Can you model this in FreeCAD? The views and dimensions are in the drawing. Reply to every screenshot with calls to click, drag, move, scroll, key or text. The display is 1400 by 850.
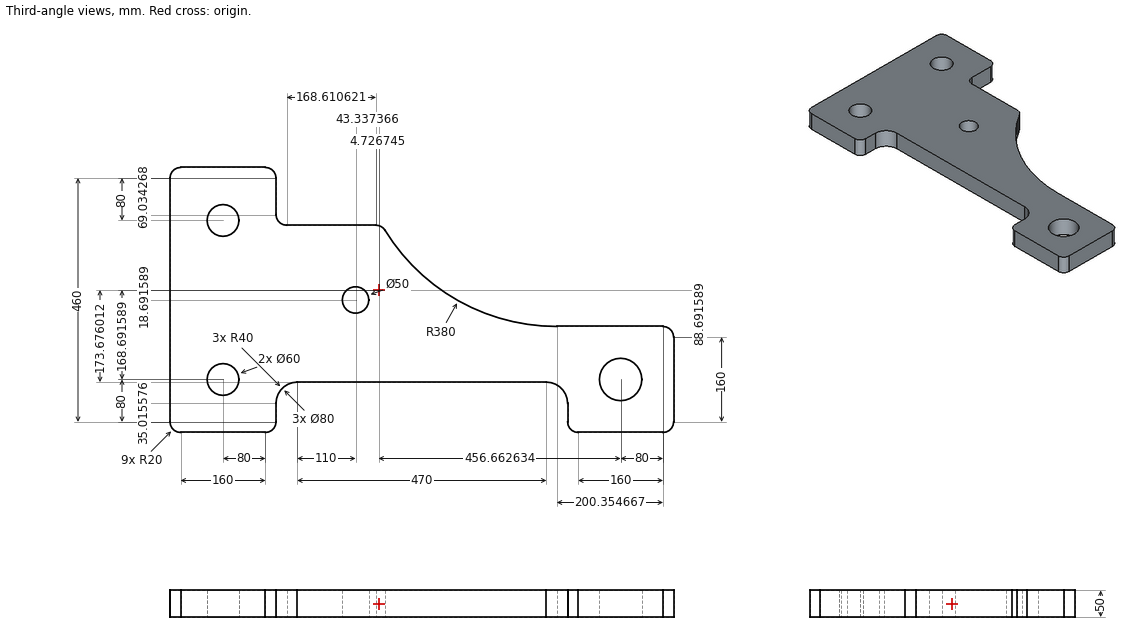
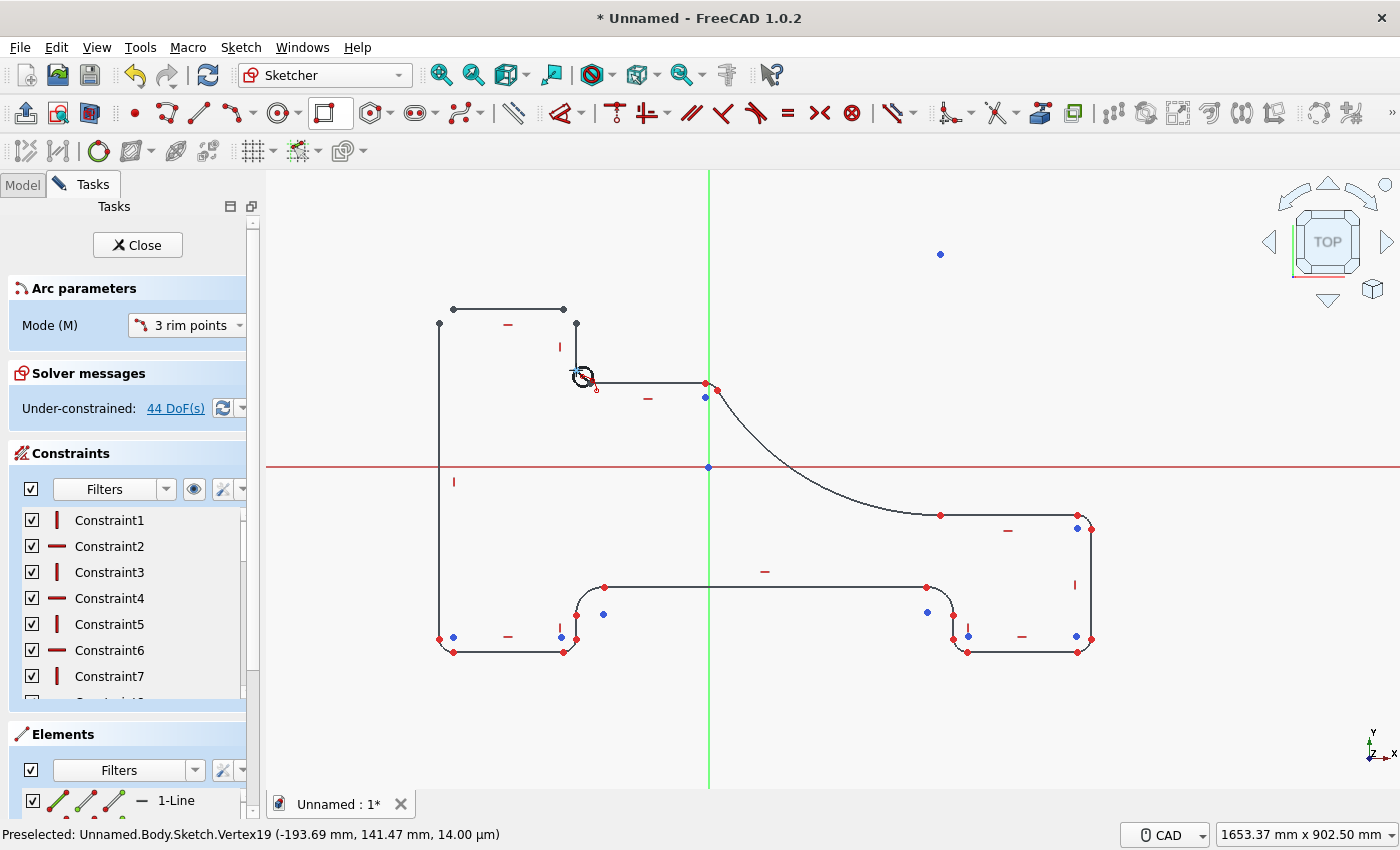
scroll(580, 379, up, 7)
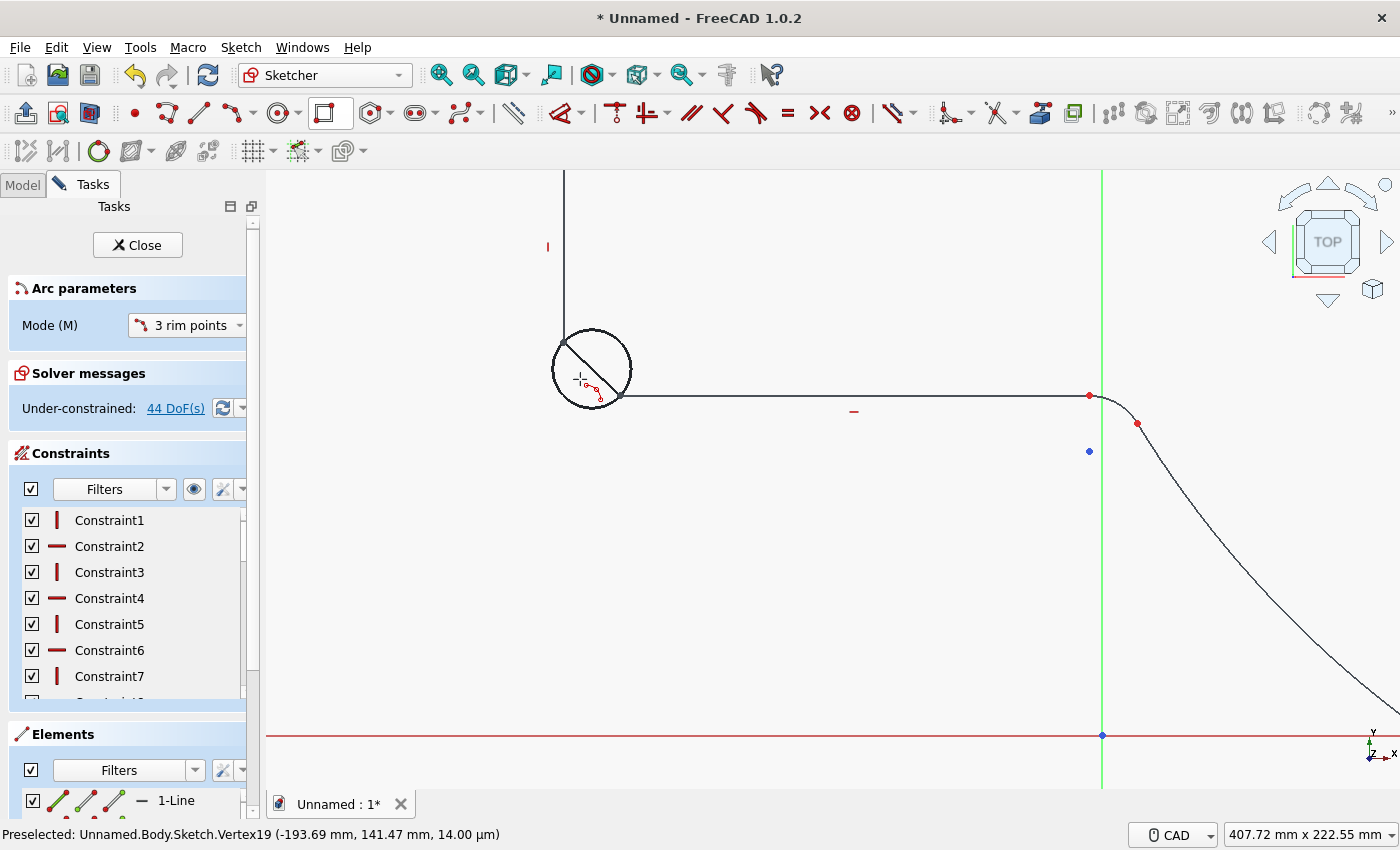
click(581, 379)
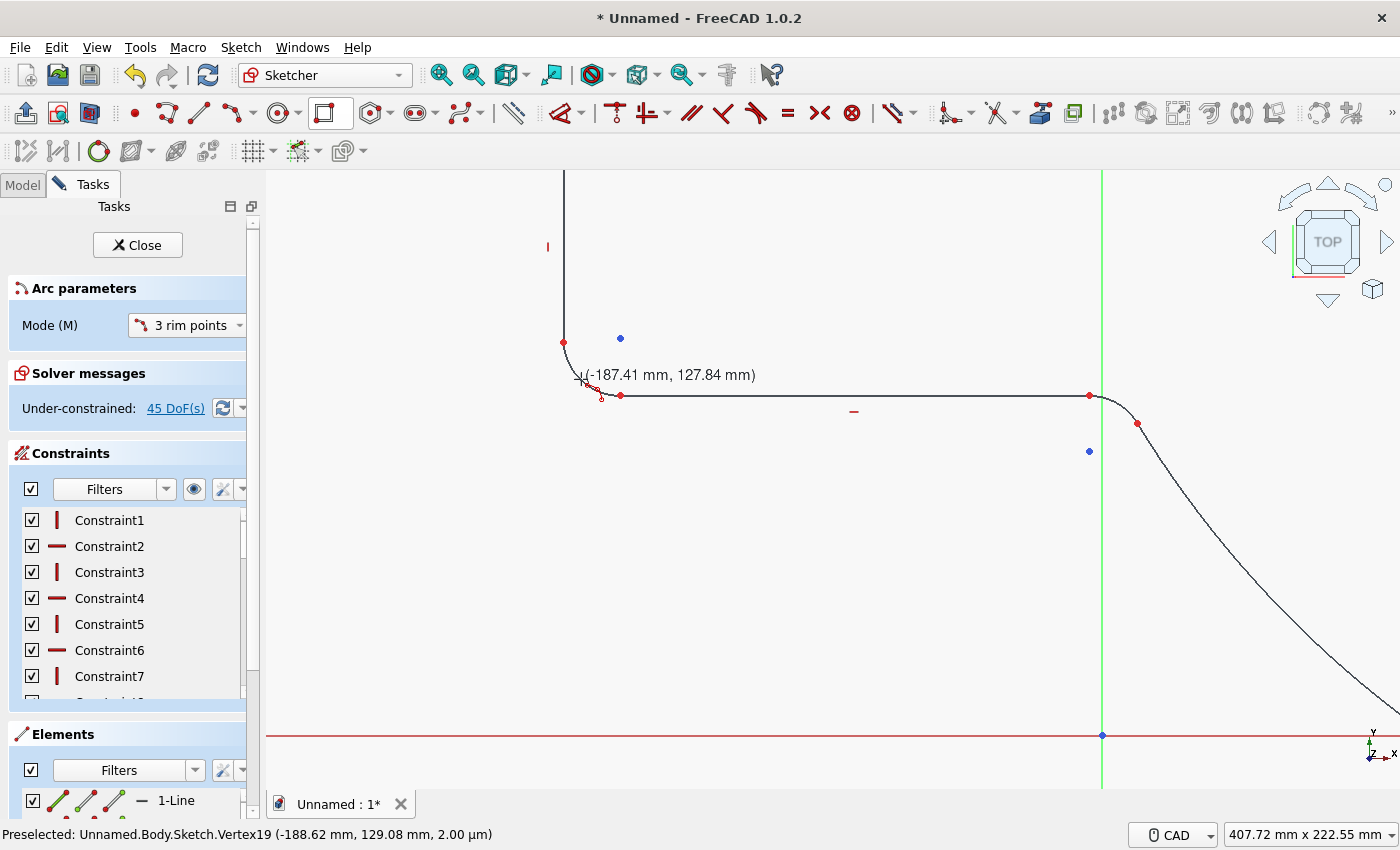
scroll(580, 379, down, 7)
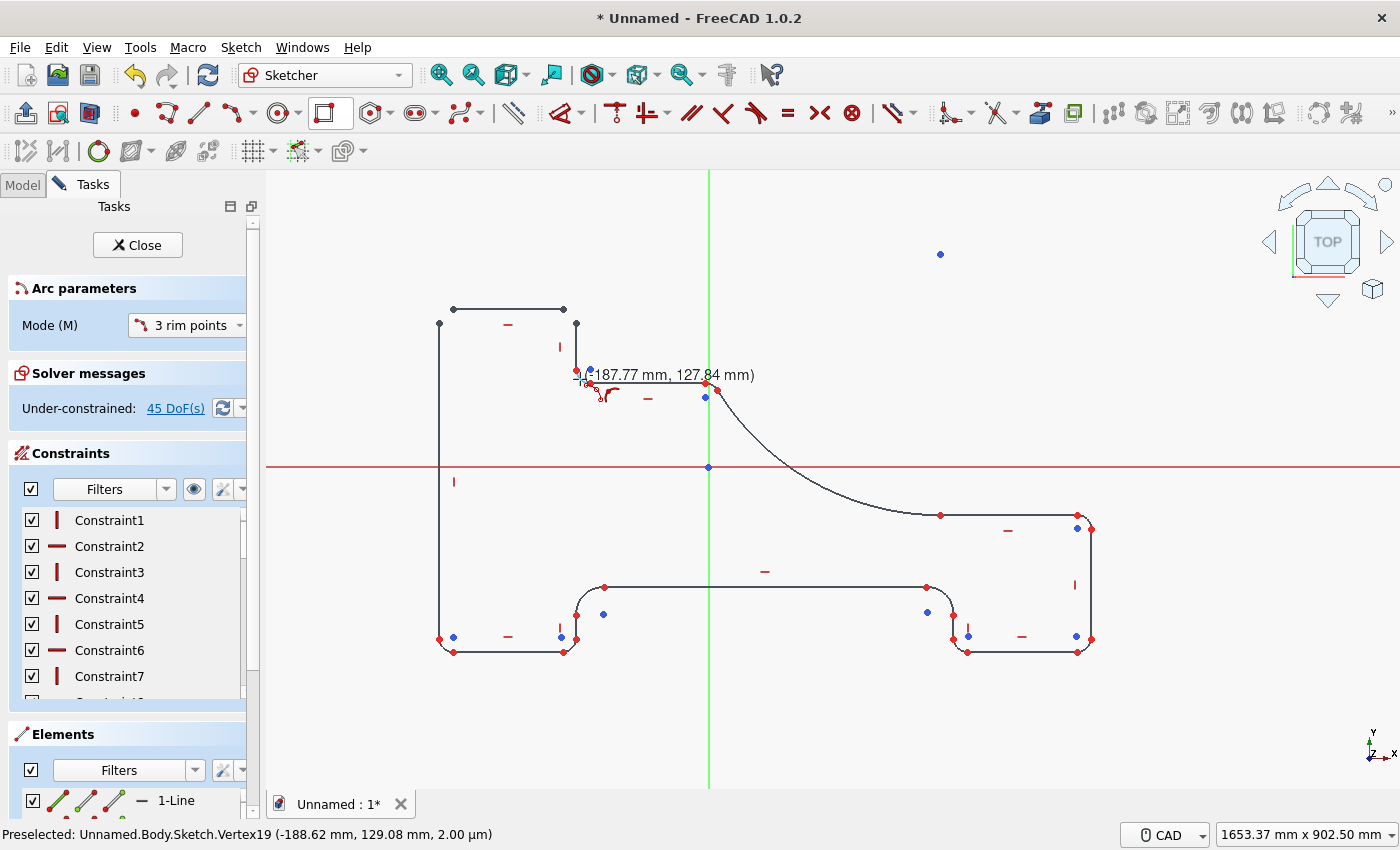
click(576, 323)
click(563, 309)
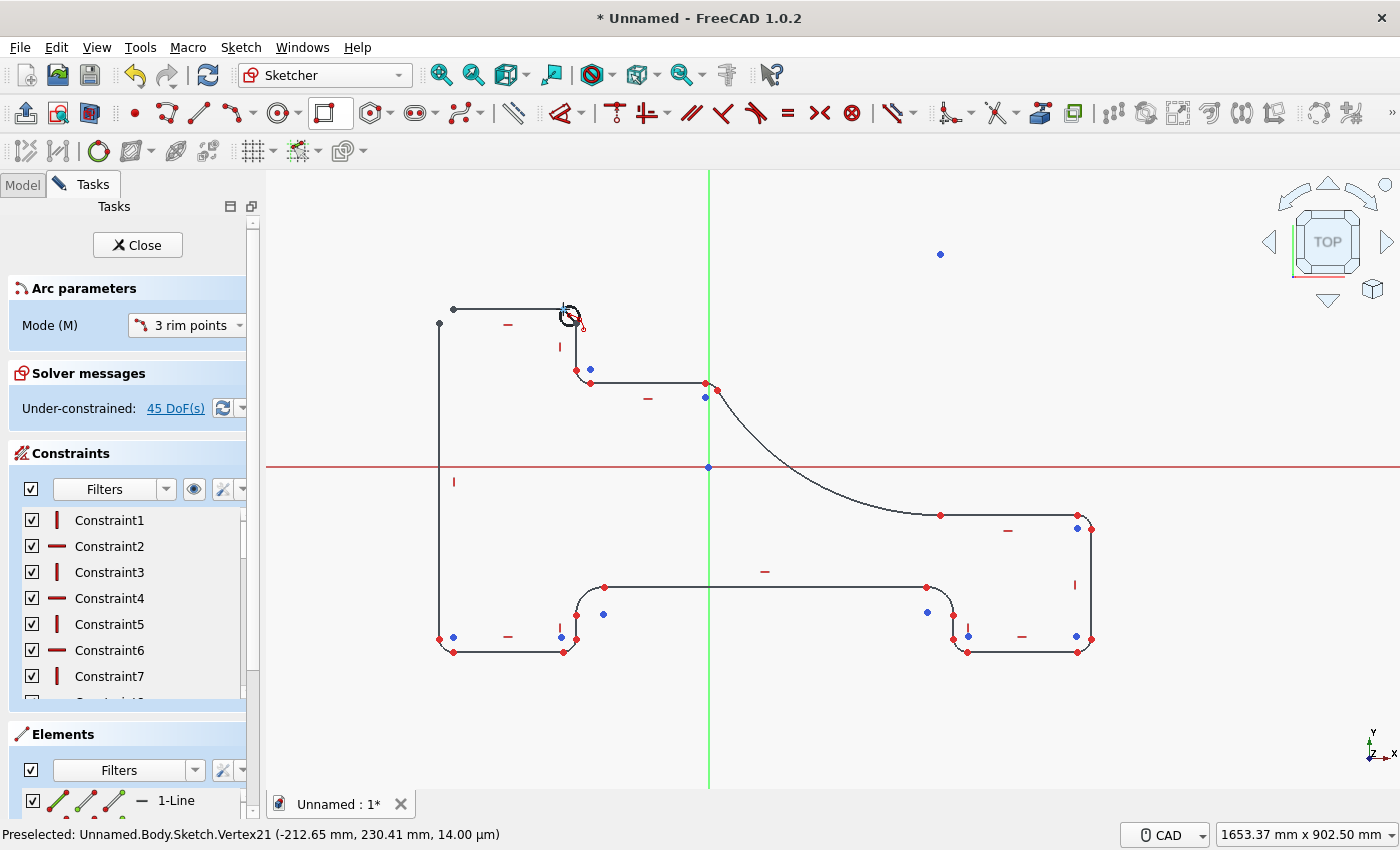
scroll(572, 313, up, 7)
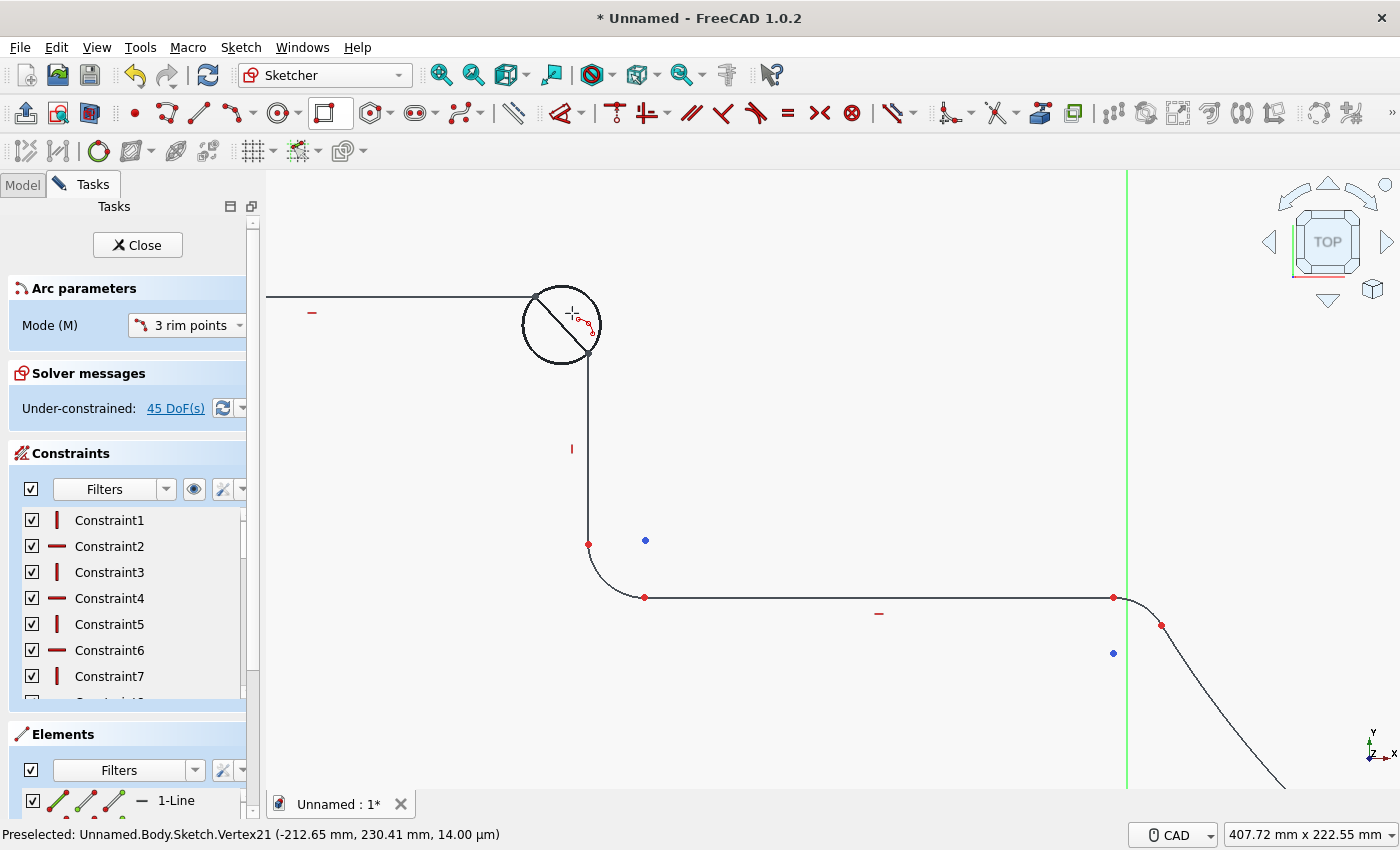
click(573, 310)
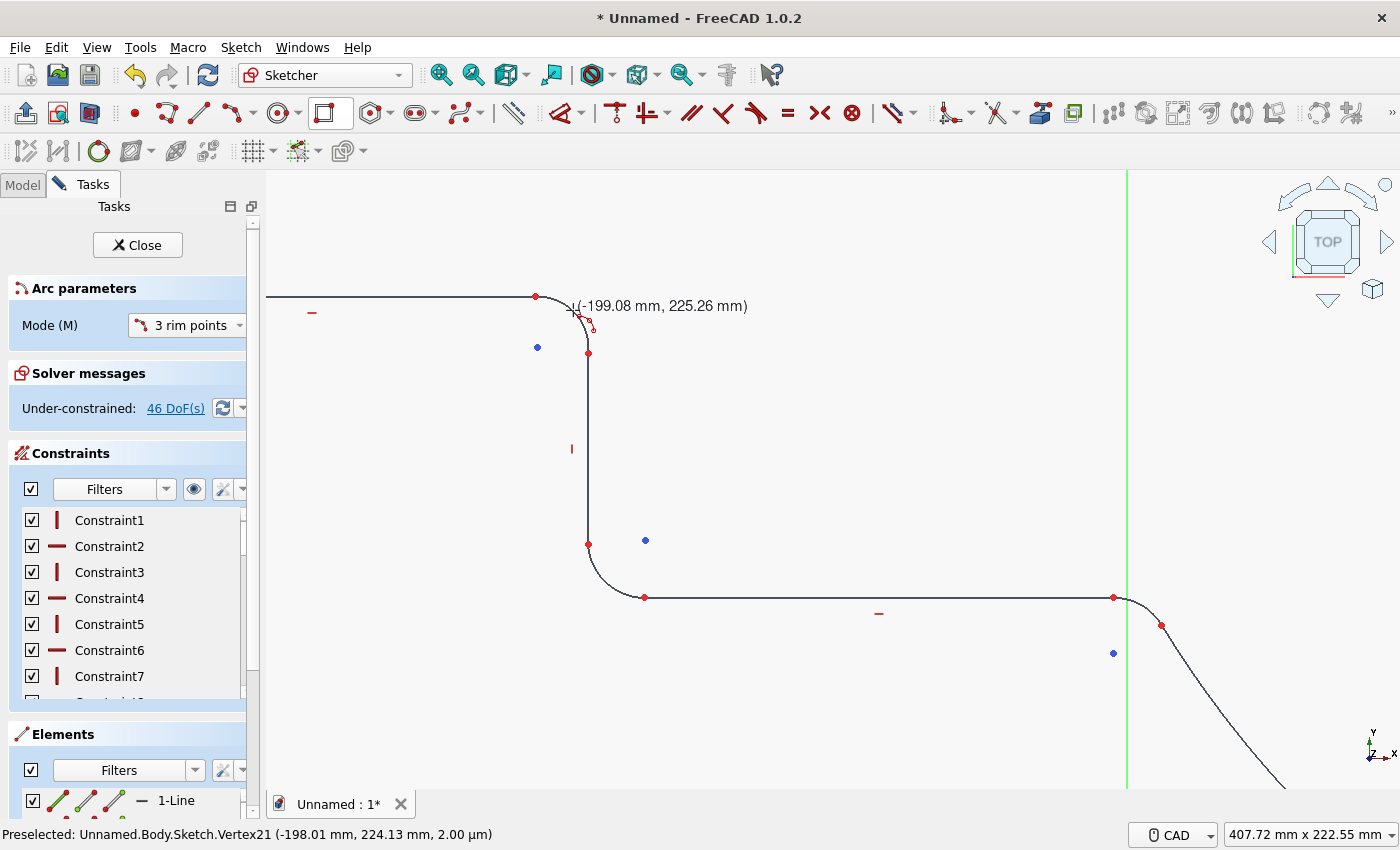
scroll(572, 313, down, 7)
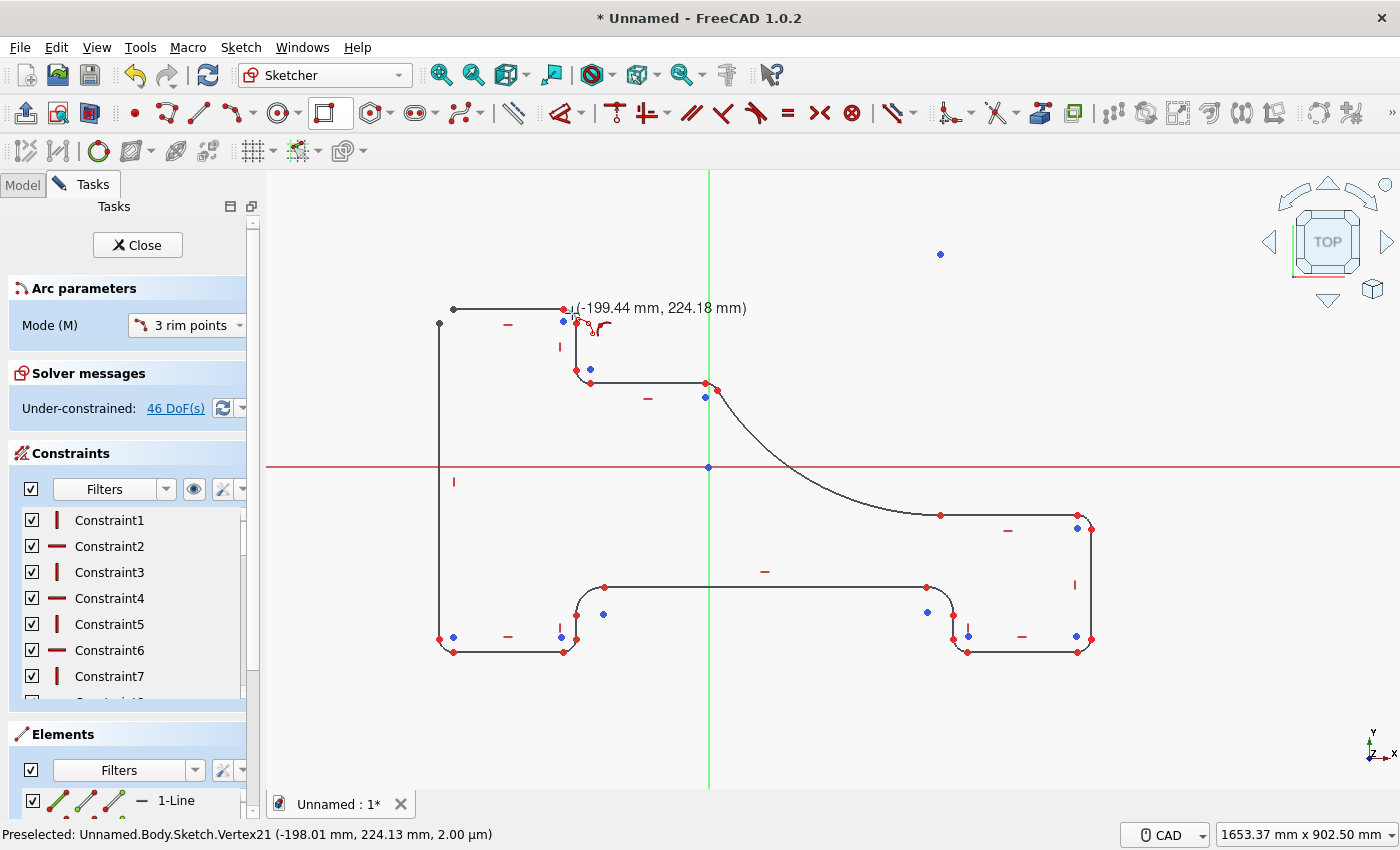
click(453, 309)
click(439, 323)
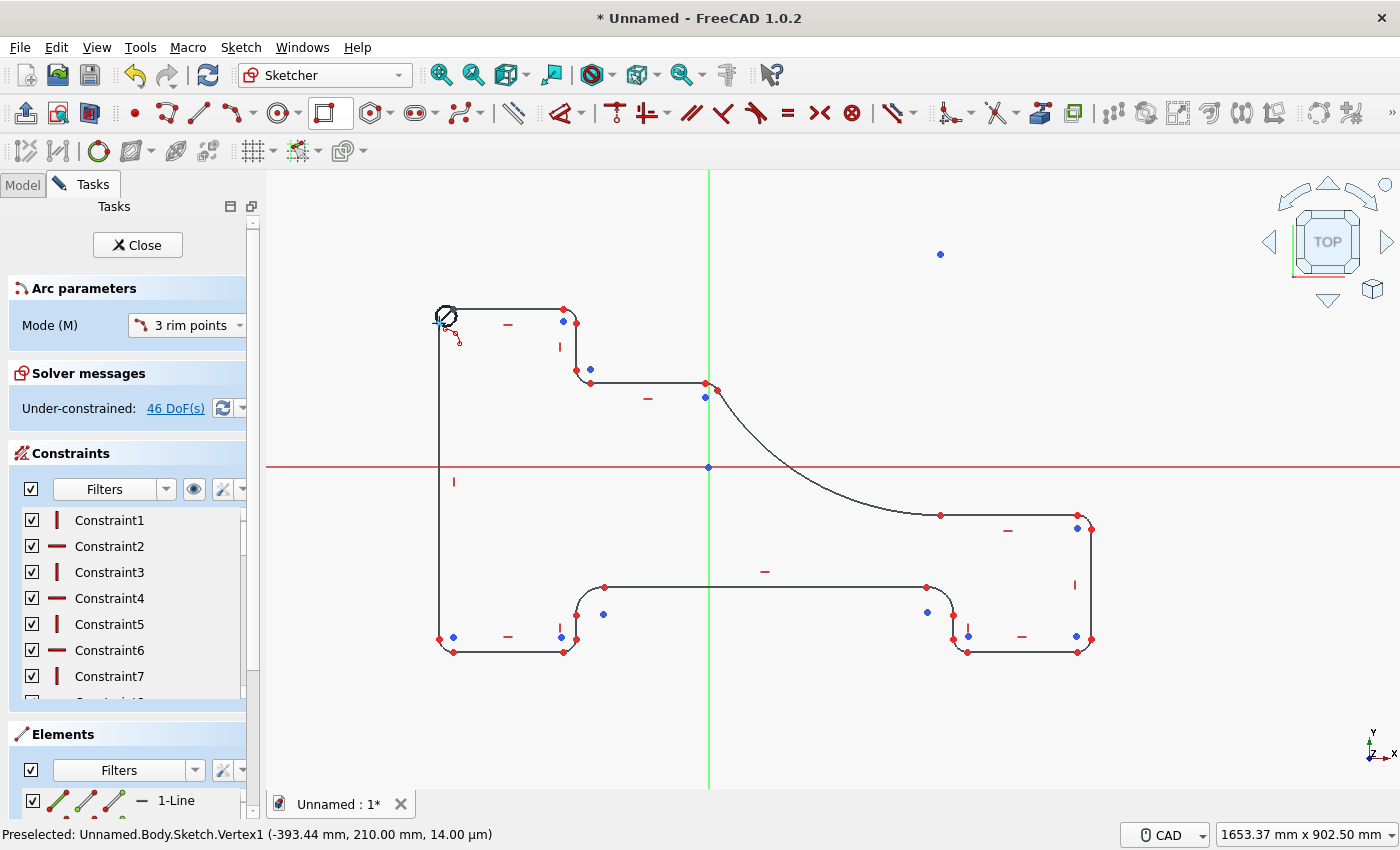
scroll(443, 313, up, 7)